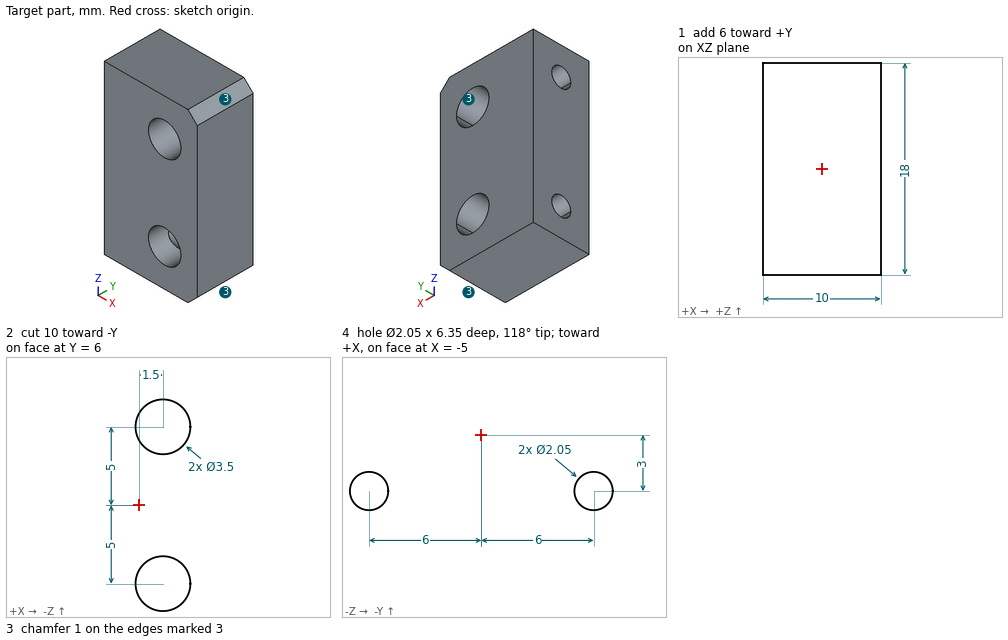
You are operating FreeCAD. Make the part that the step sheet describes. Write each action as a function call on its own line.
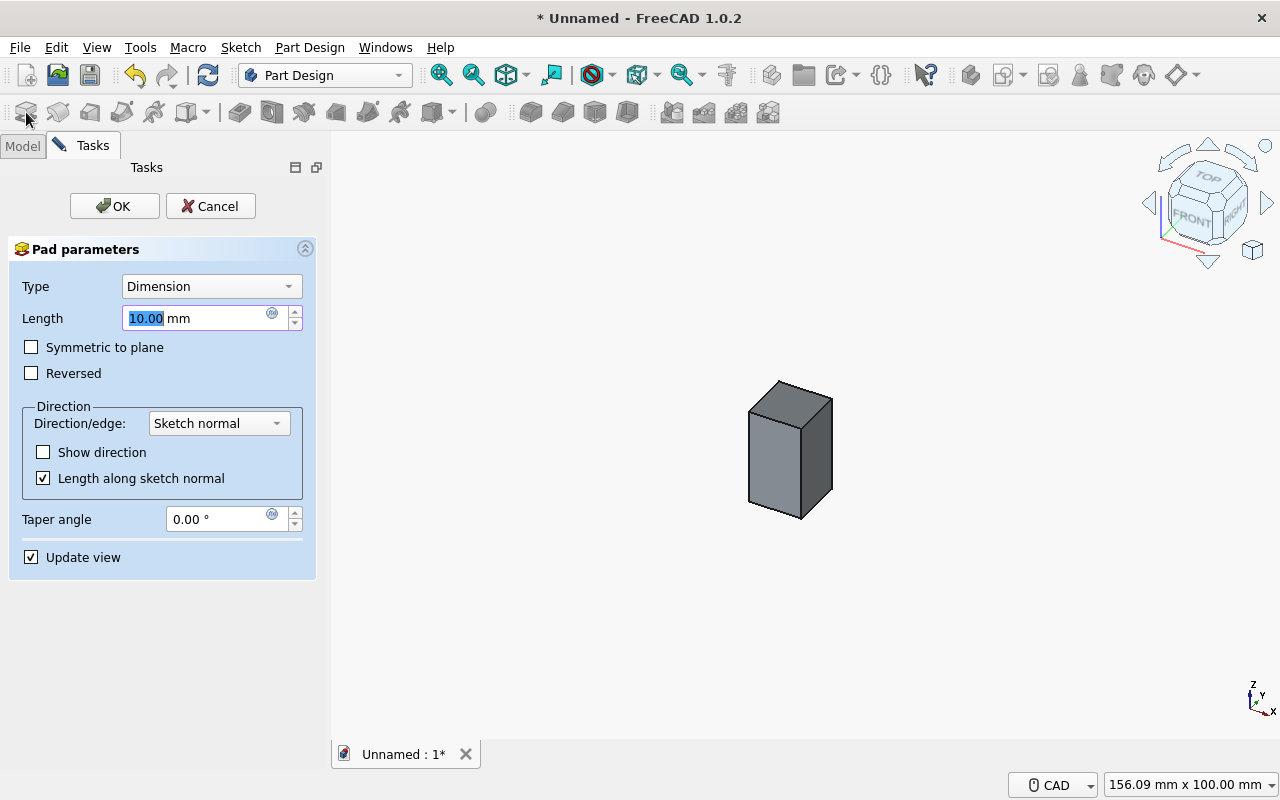
text(6)
key(Tab)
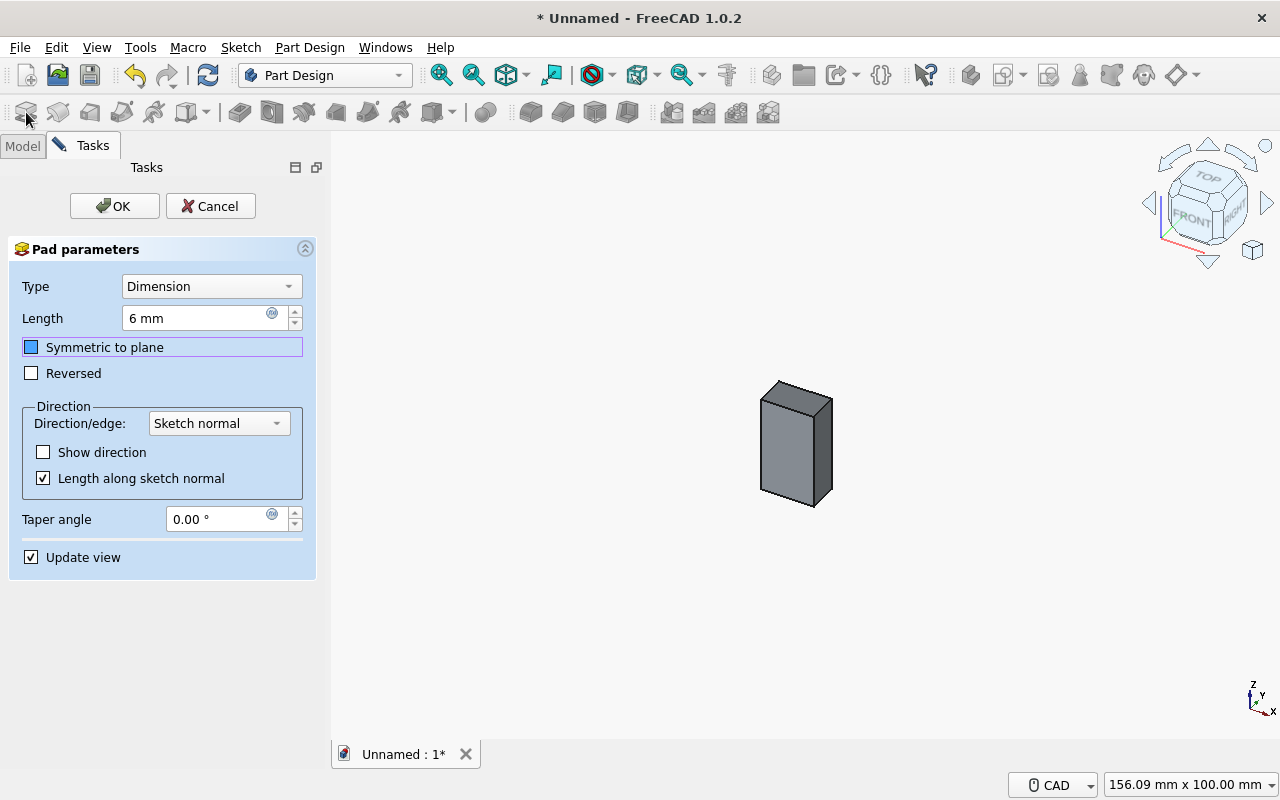
click(30, 373)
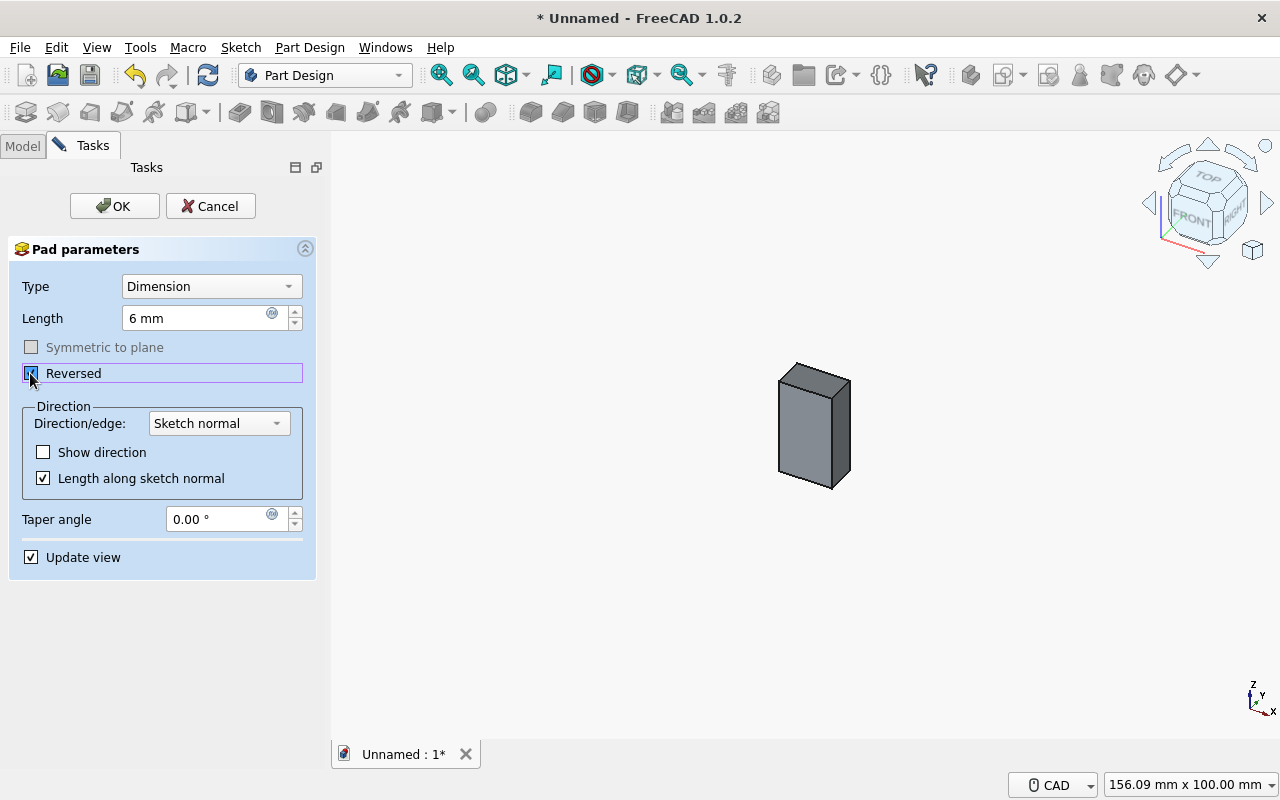
click(115, 206)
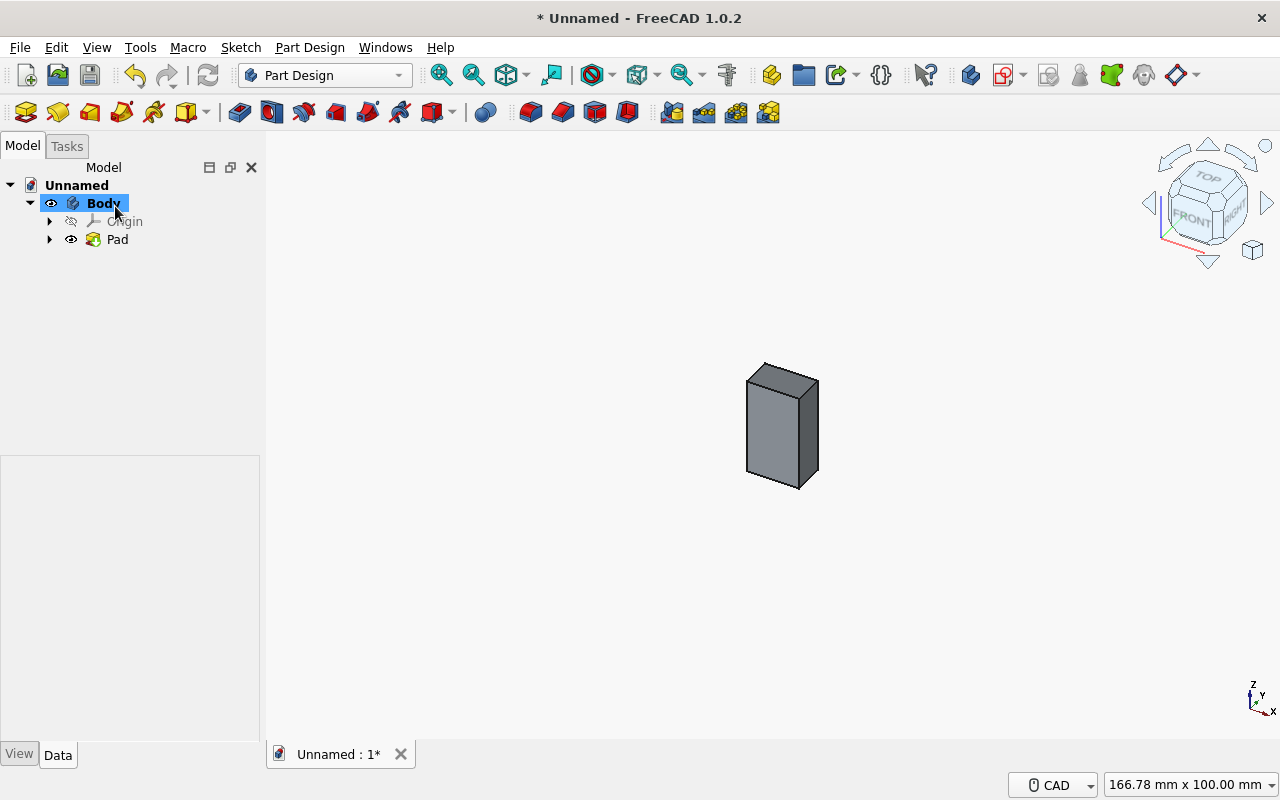
key(v)
key(f)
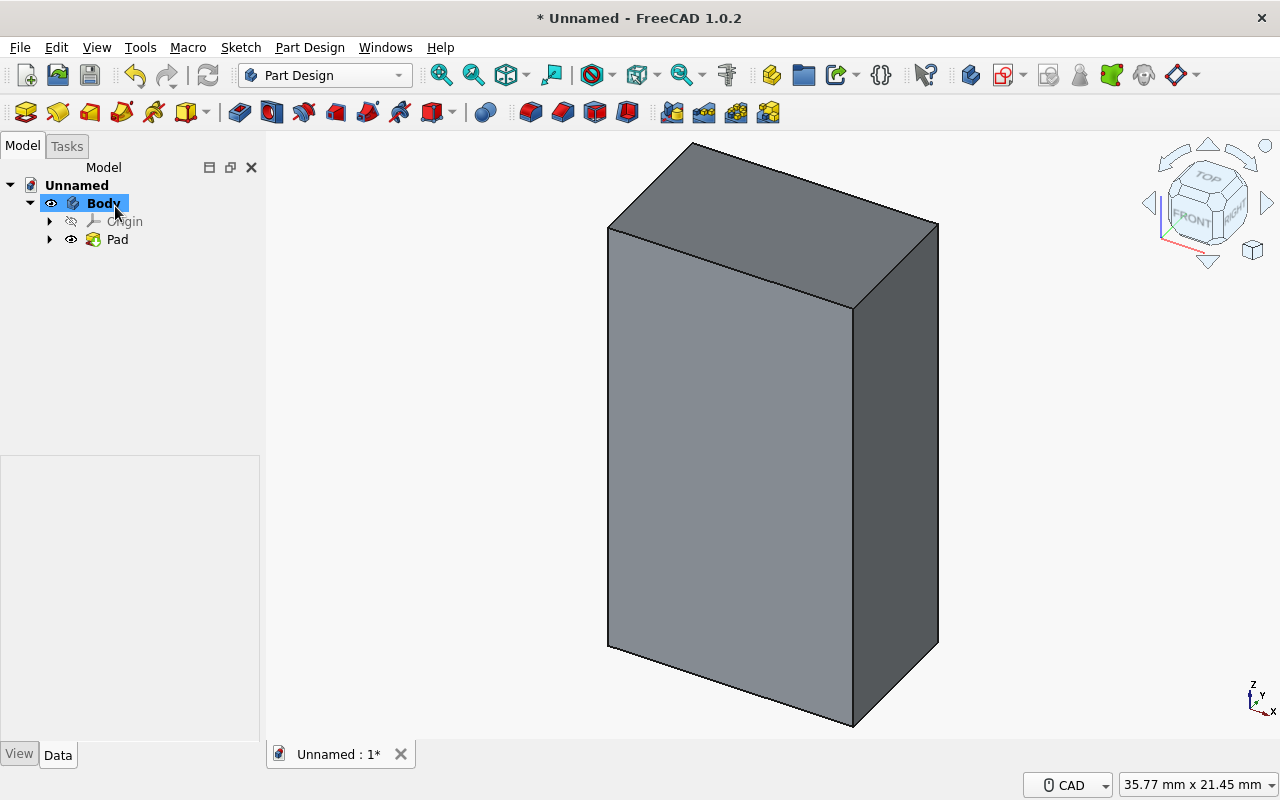
key(4)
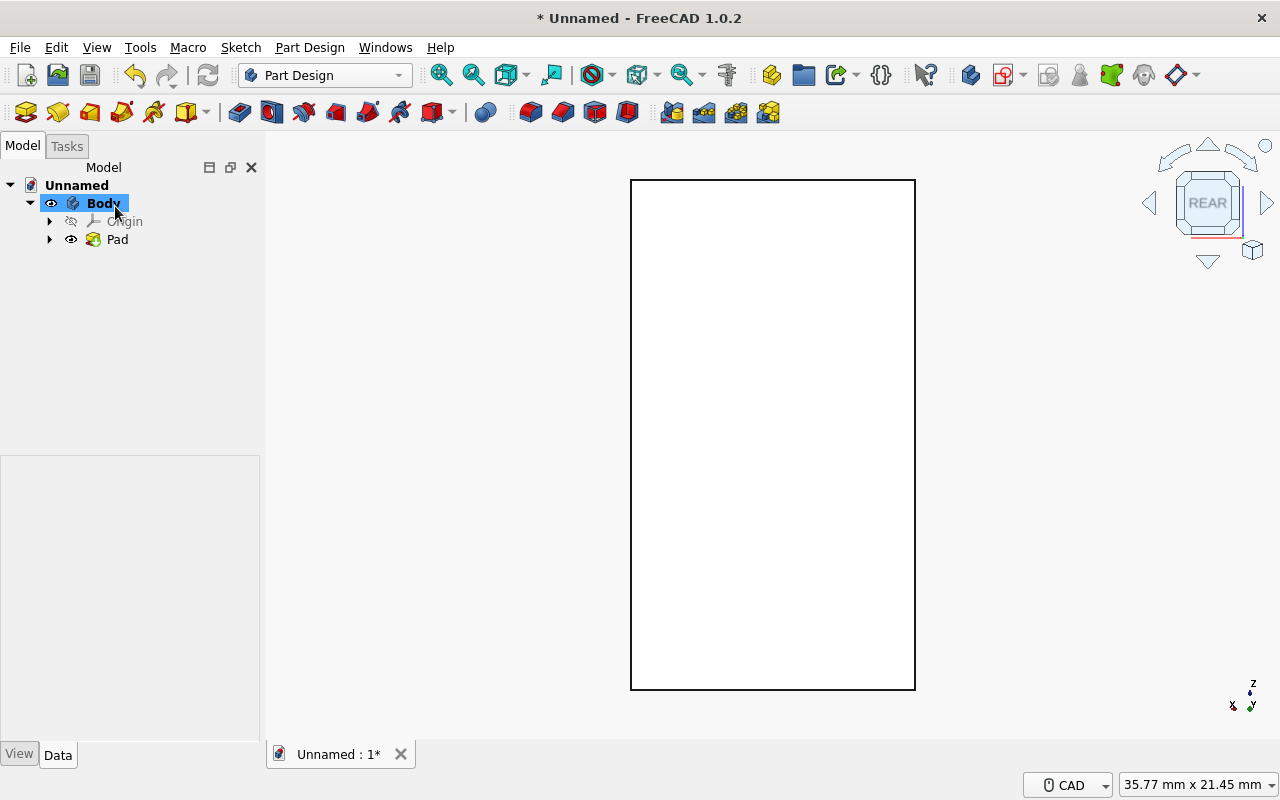
click(773, 361)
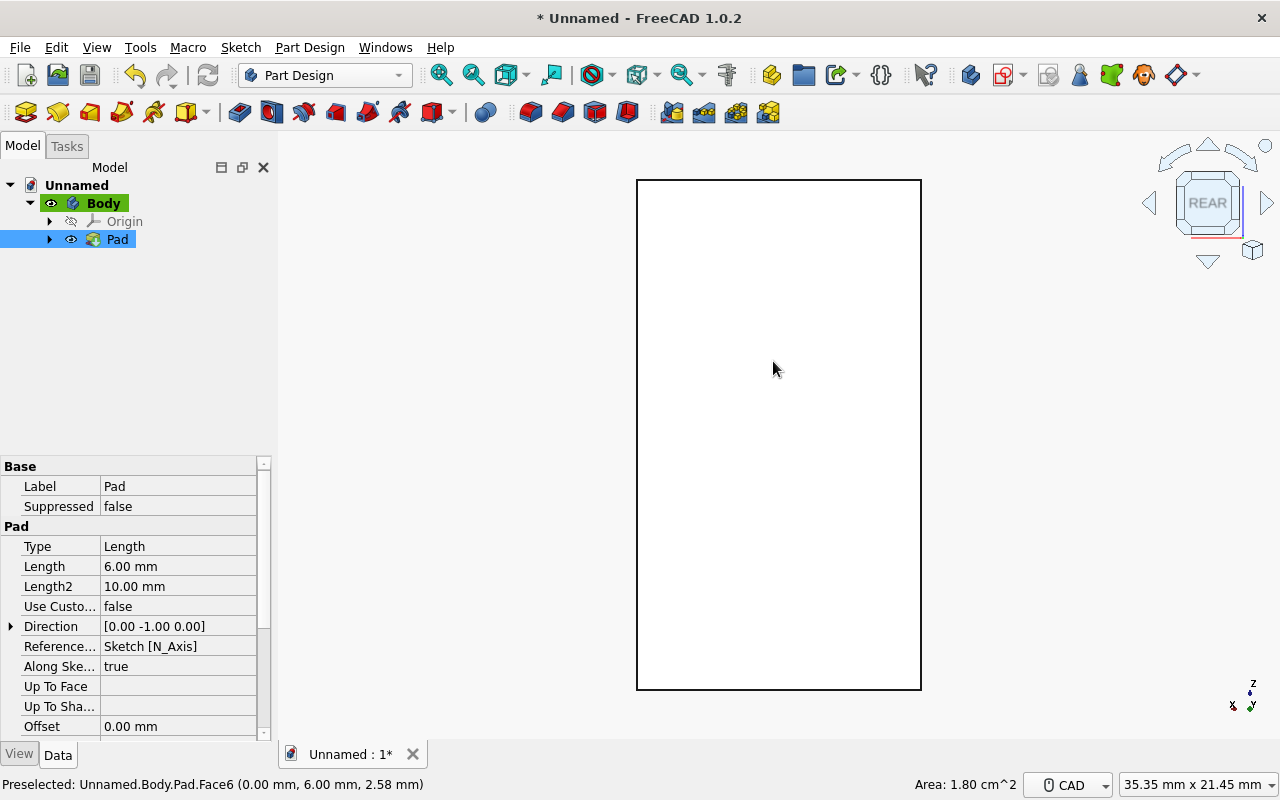
click(1004, 76)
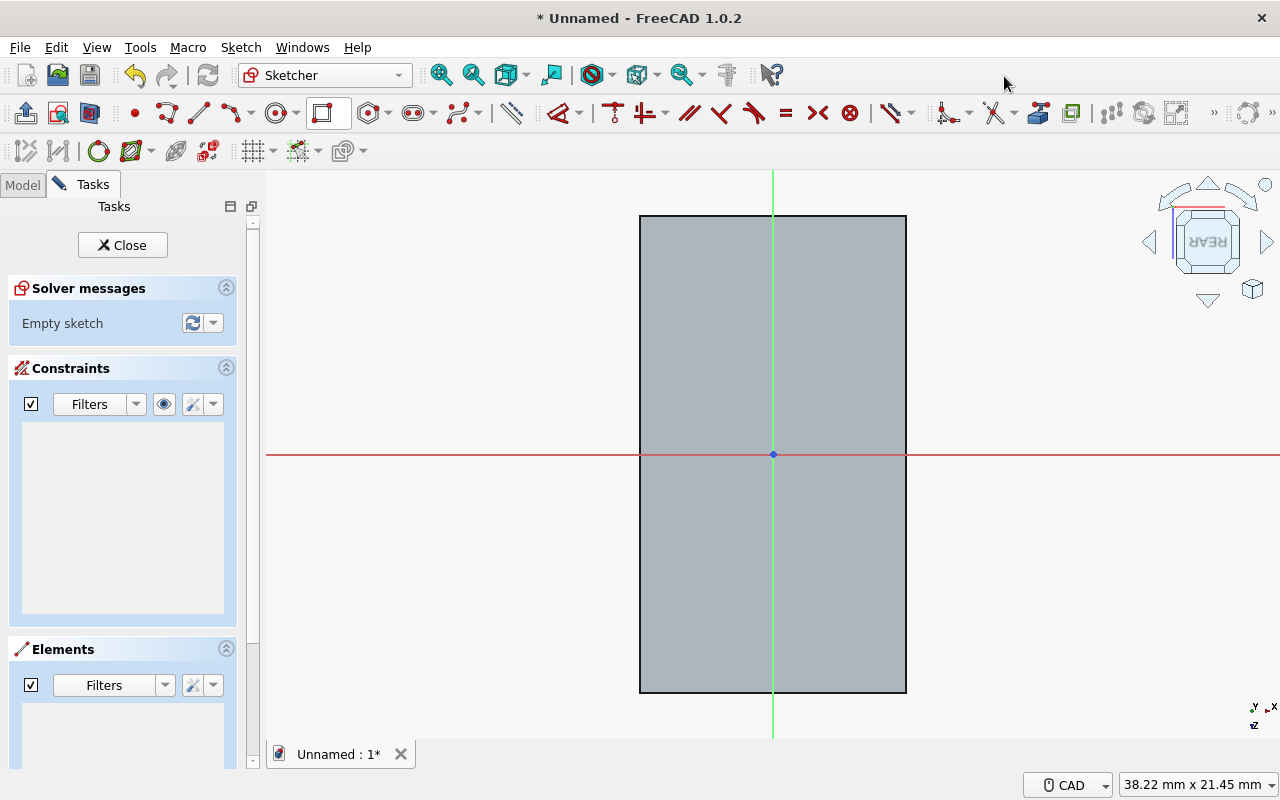
key(g)
key(c)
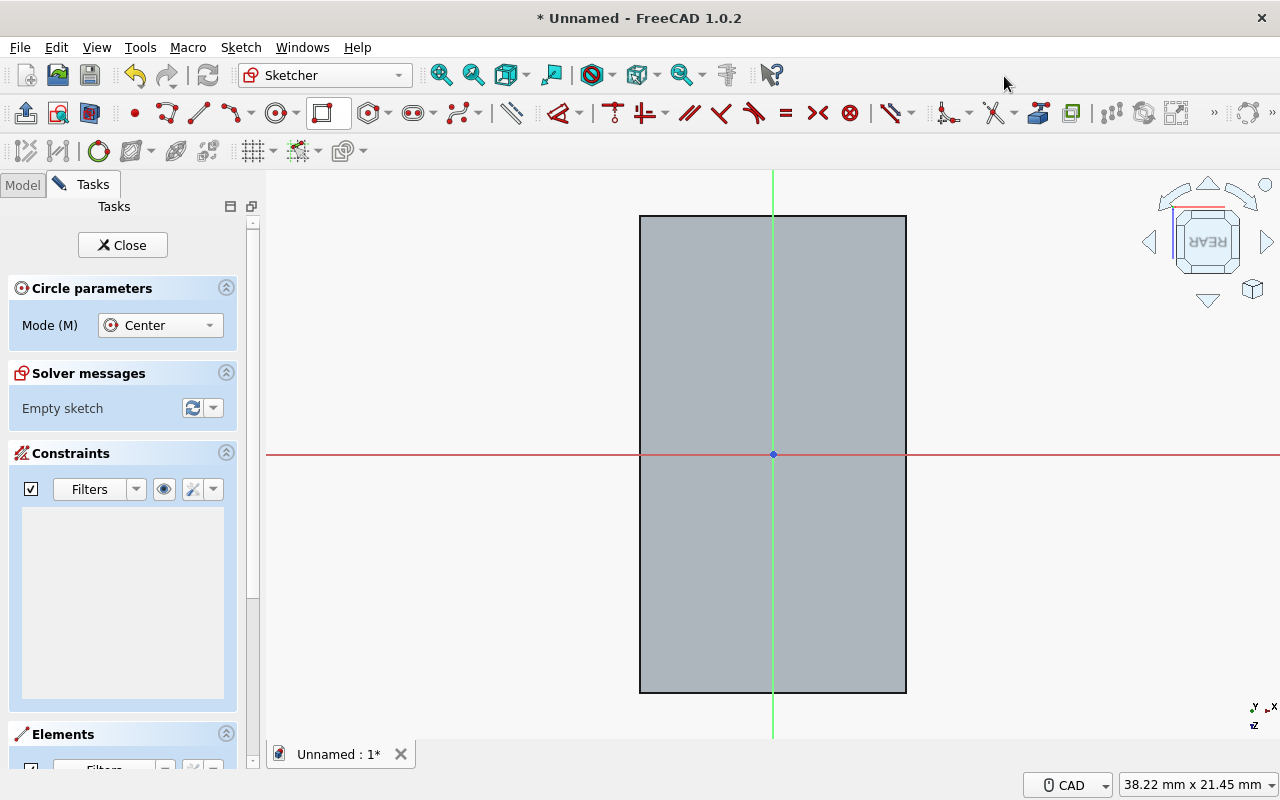
click(813, 322)
move(846, 289)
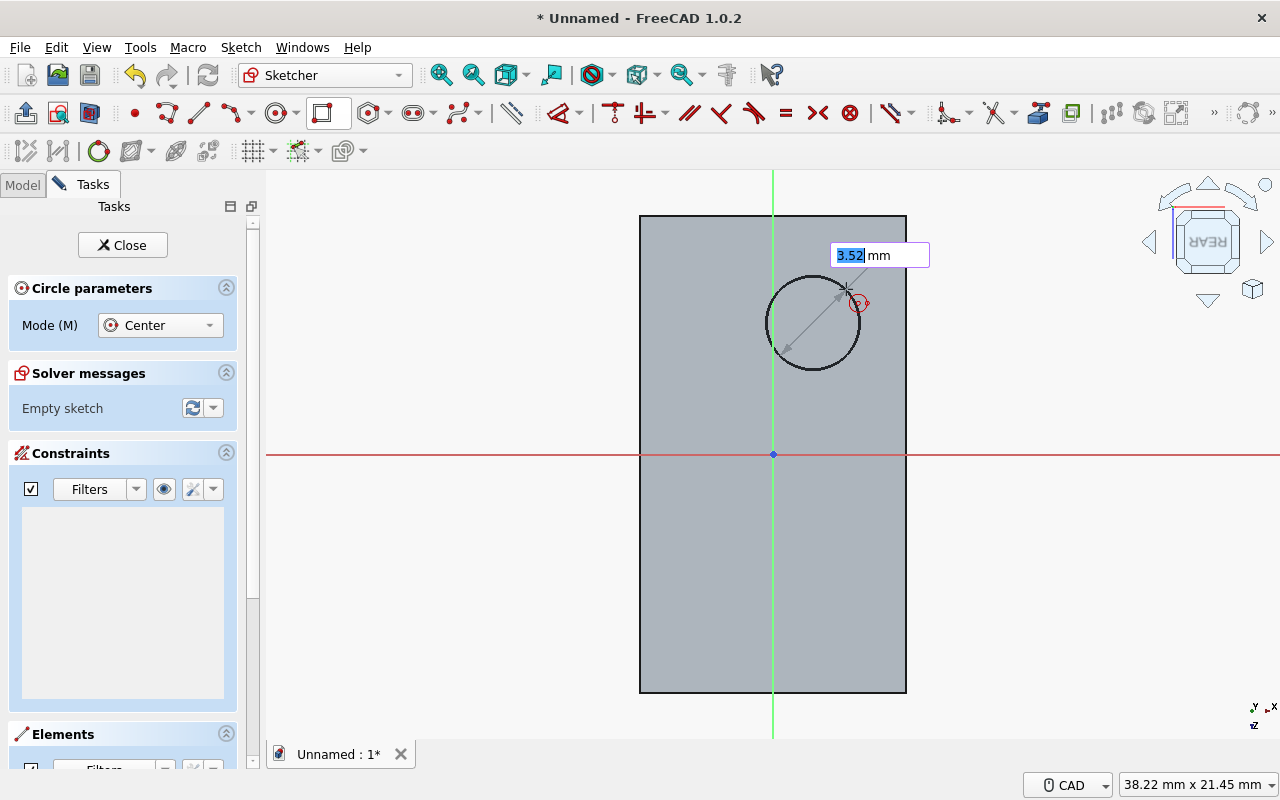
text(3.5)
key(Return)